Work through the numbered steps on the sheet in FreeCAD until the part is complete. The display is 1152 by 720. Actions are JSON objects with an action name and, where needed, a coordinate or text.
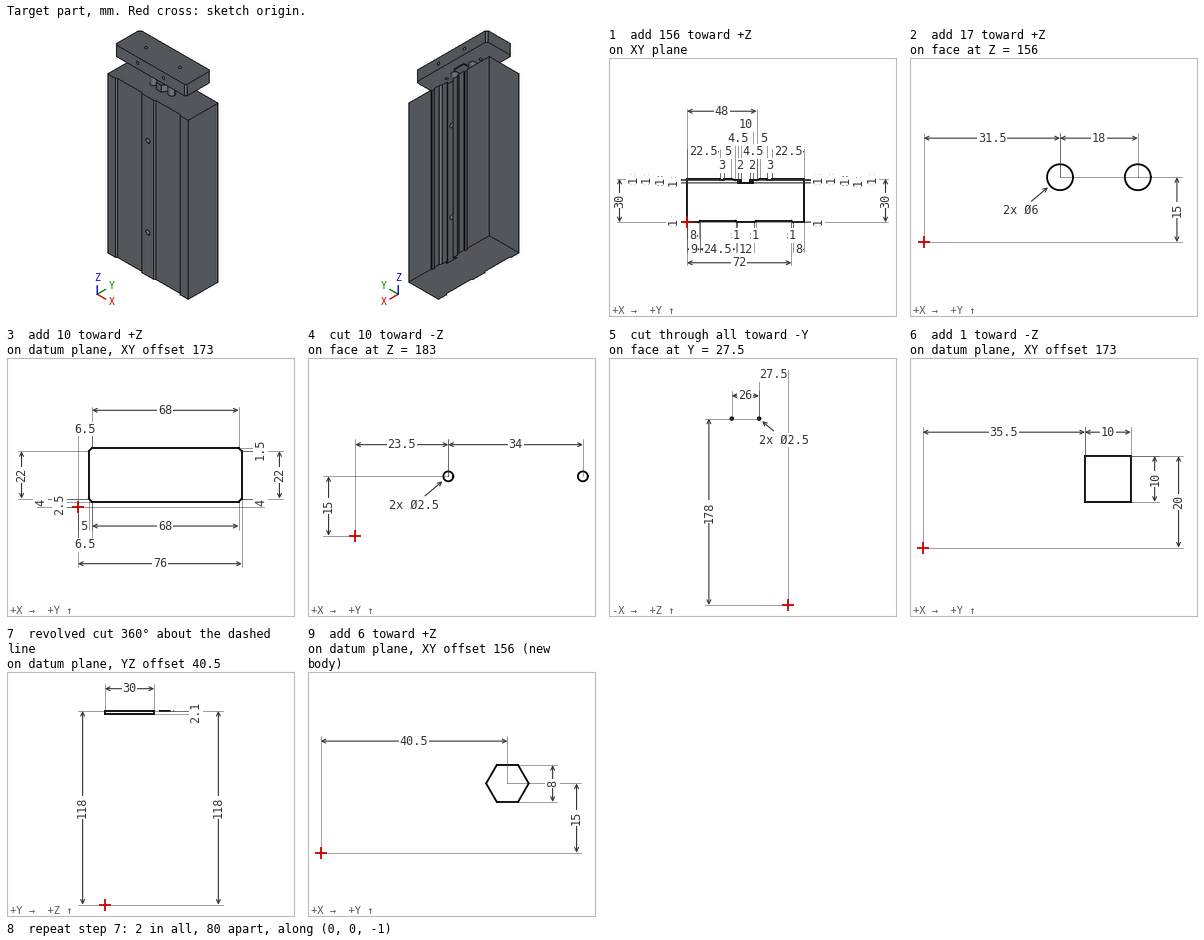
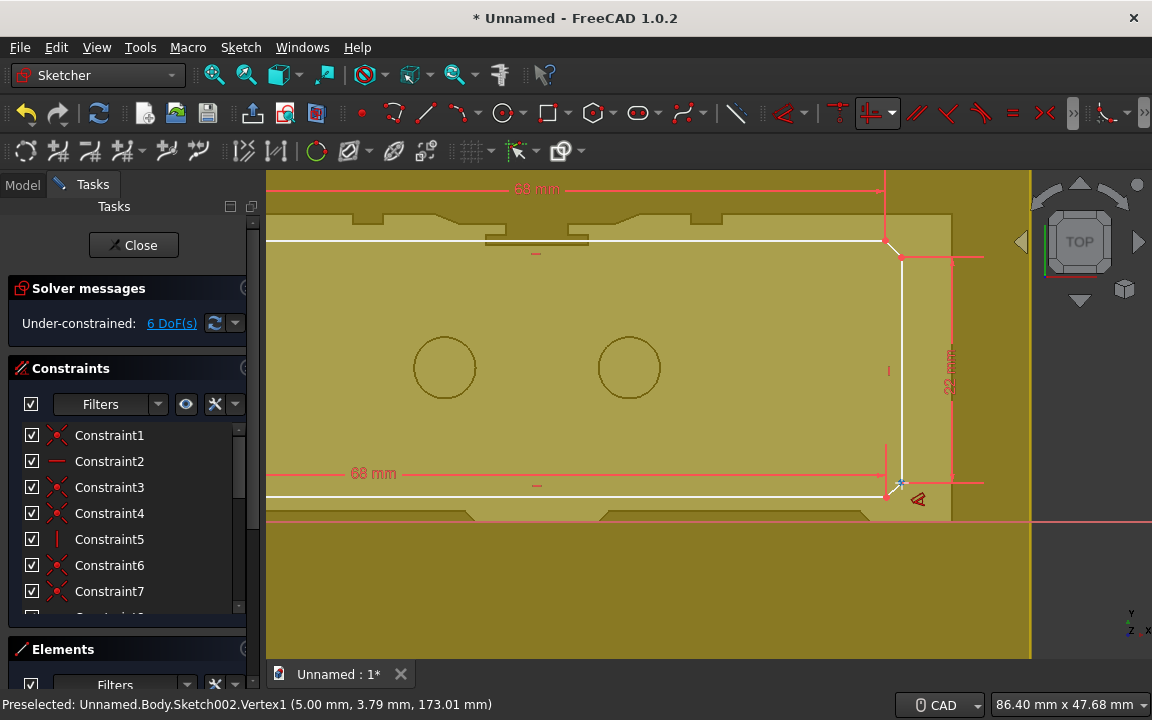
{"action": "left_click", "coordinate": [902, 483]}
{"action": "left_click", "coordinate": [936, 502]}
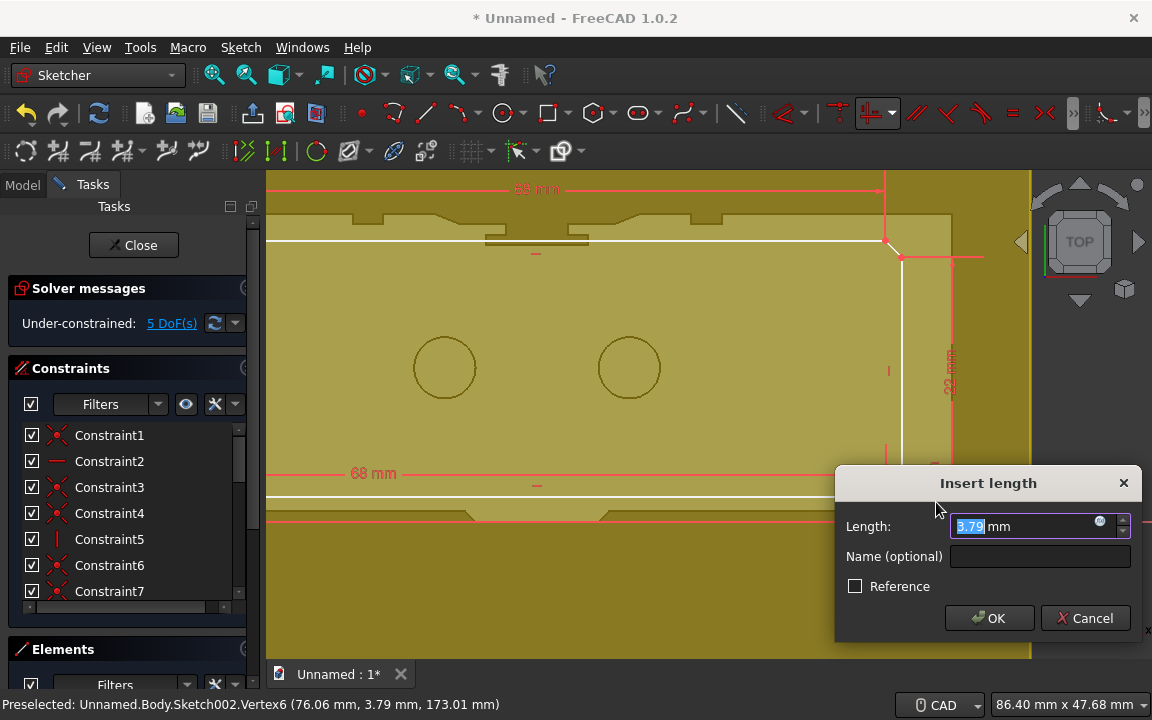
{"action": "type", "text": "4"}
{"action": "key", "text": "Return"}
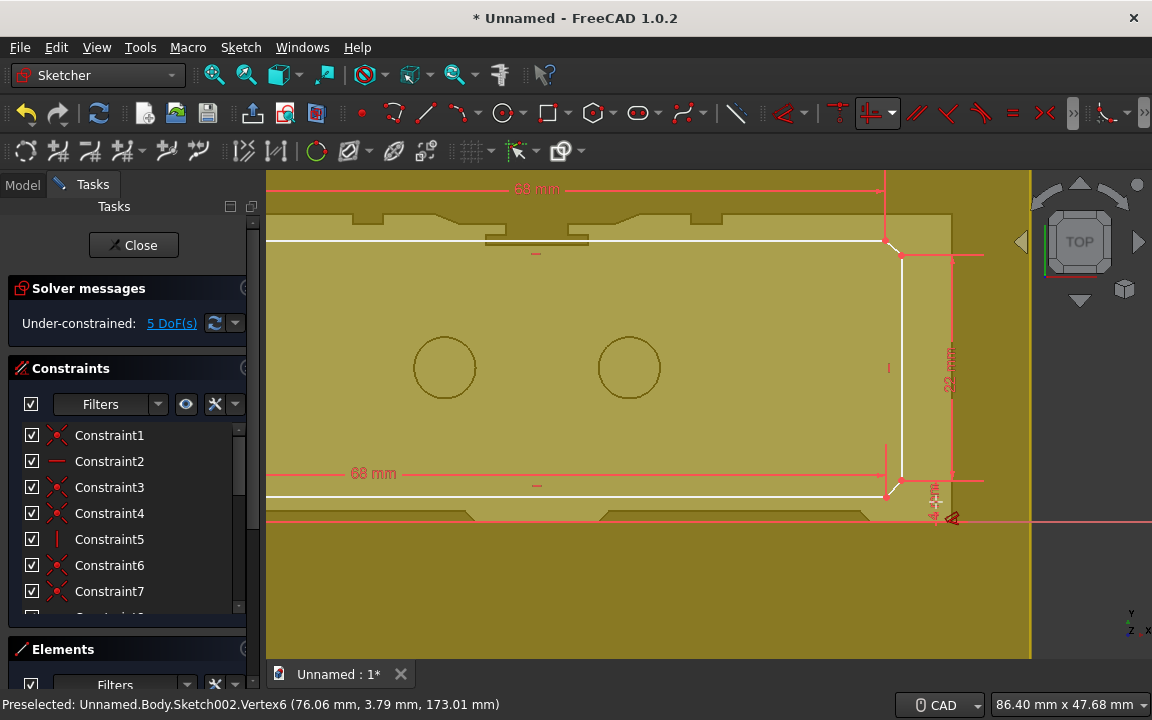
{"action": "left_click", "coordinate": [902, 481]}
{"action": "left_click", "coordinate": [598, 556]}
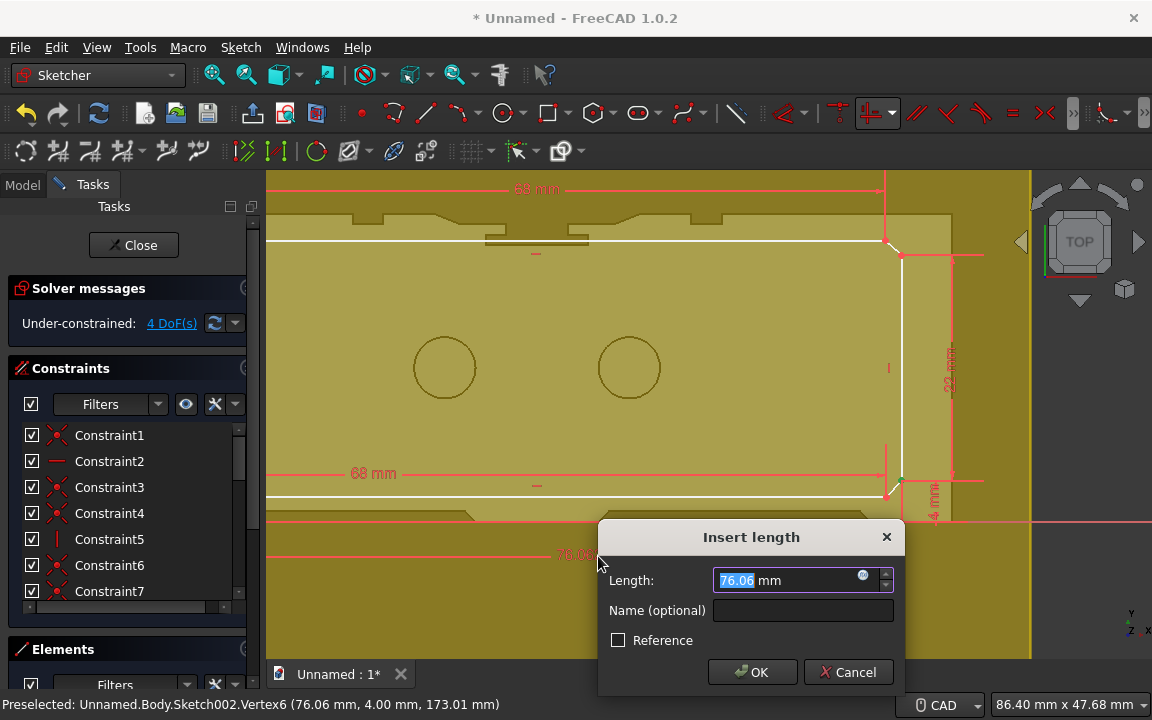
{"action": "type", "text": "76"}
{"action": "key", "text": "Return"}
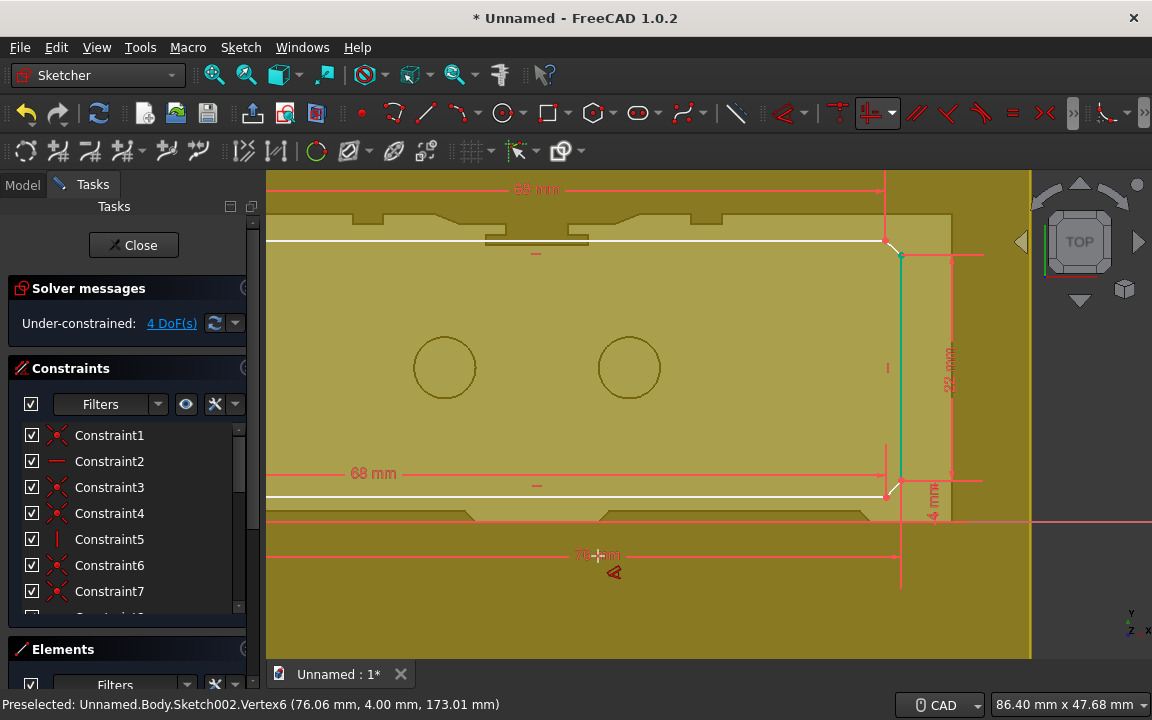
{"action": "scroll", "coordinate": [903, 483], "scroll_direction": "down", "scroll_amount": 2}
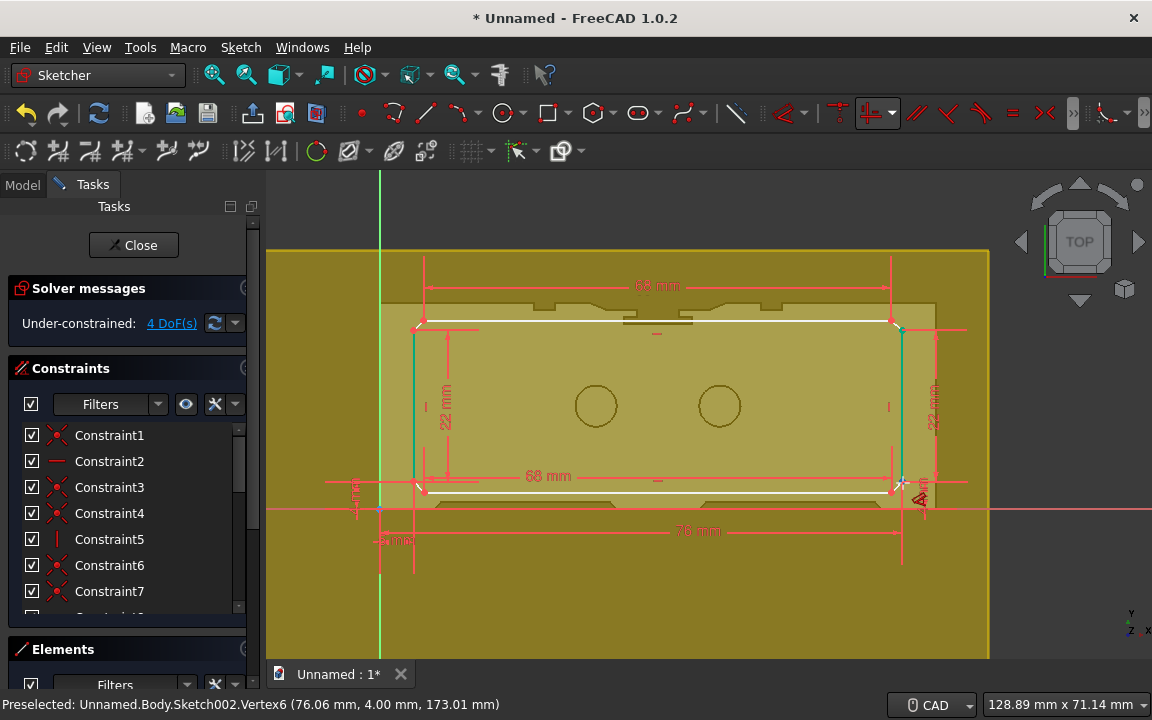
{"action": "left_click", "coordinate": [424, 493]}
{"action": "left_click", "coordinate": [402, 567]}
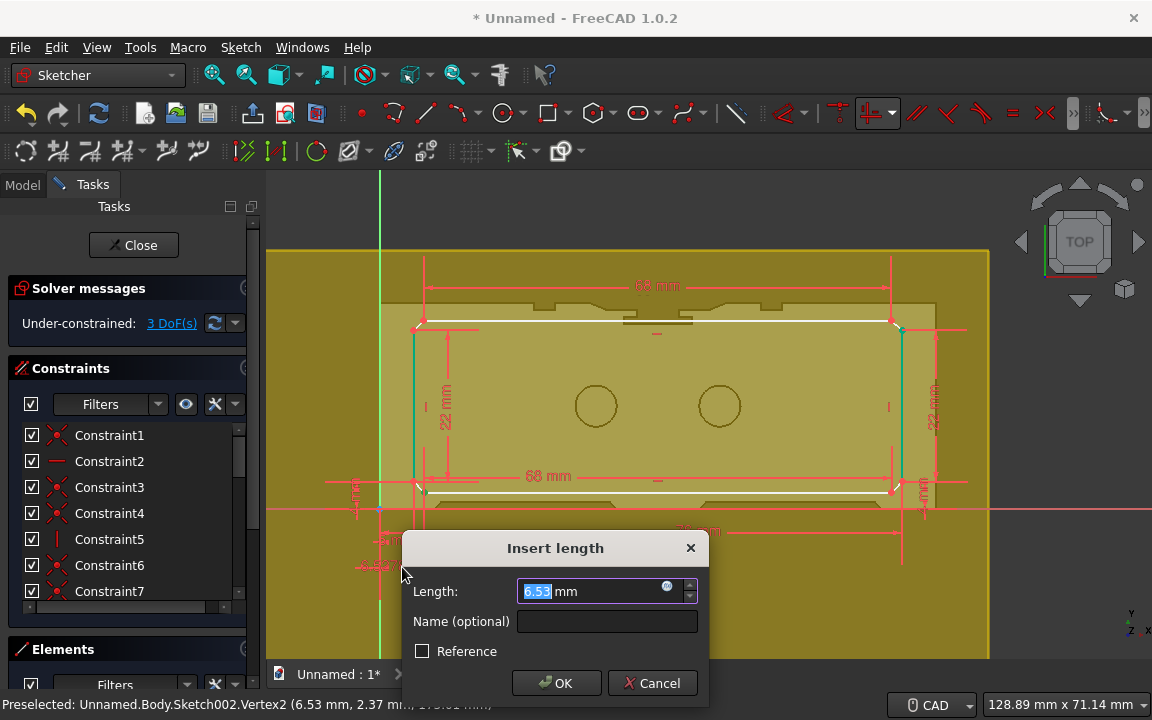
{"action": "type", "text": "6.5"}
{"action": "key", "text": "Return"}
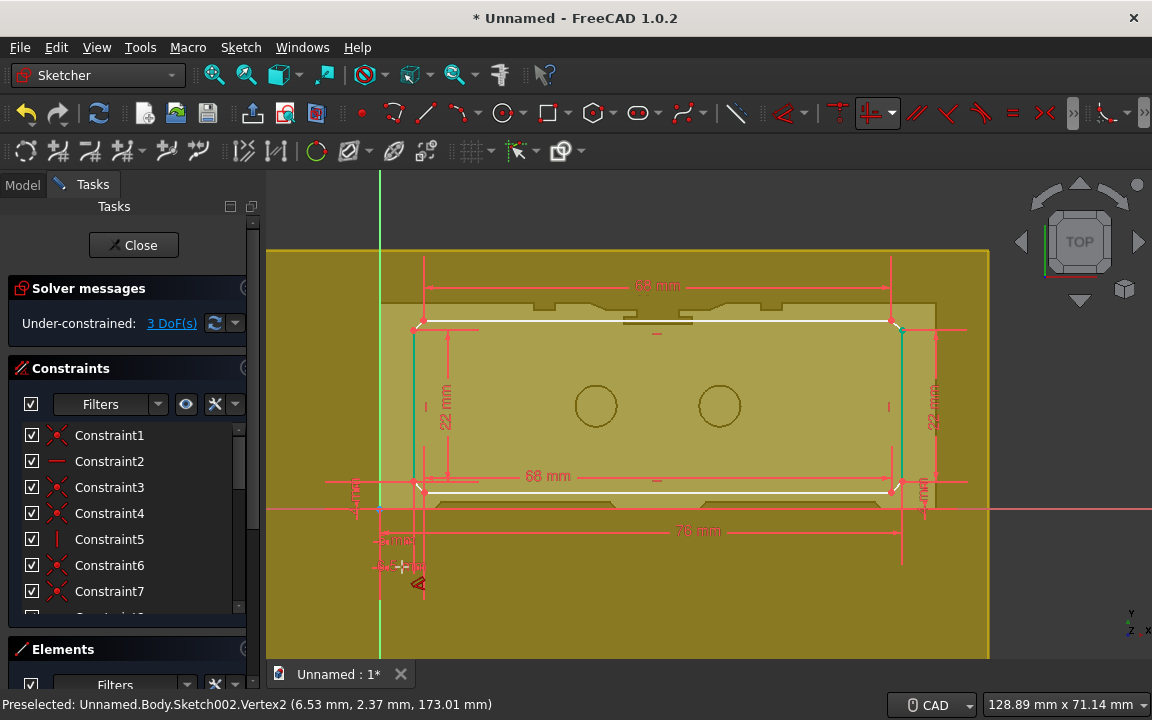
{"action": "scroll", "coordinate": [424, 493], "scroll_direction": "up", "scroll_amount": 5}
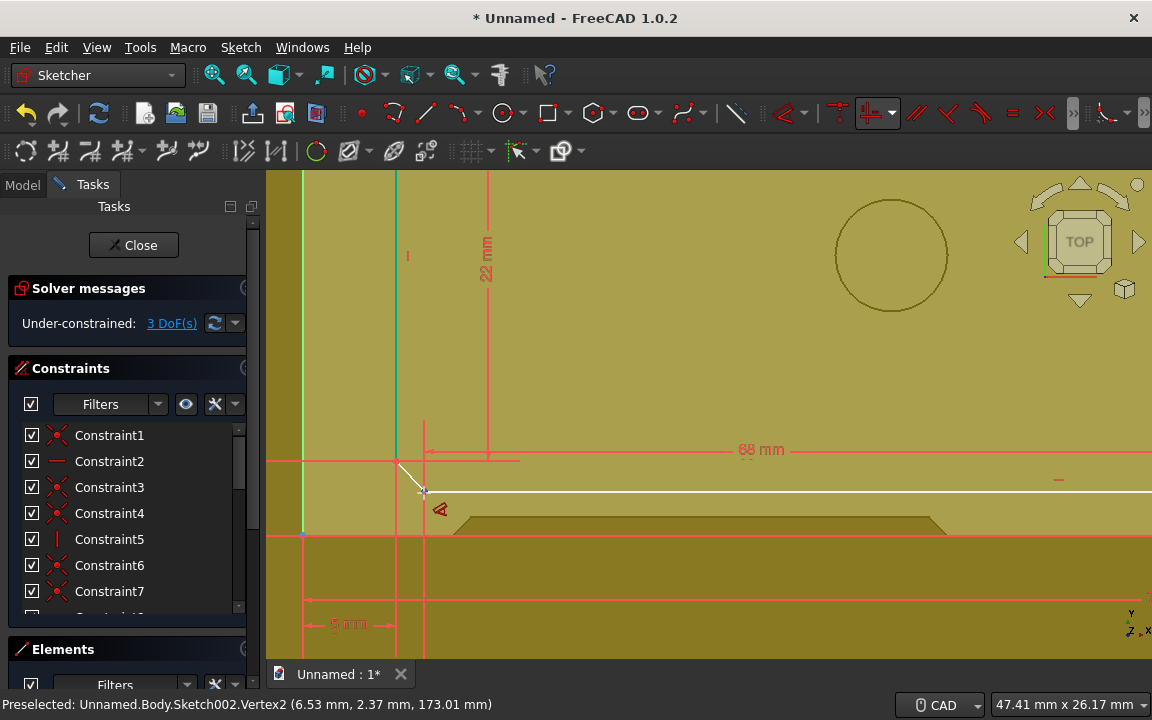
{"action": "left_click", "coordinate": [424, 492]}
{"action": "left_click", "coordinate": [458, 514]}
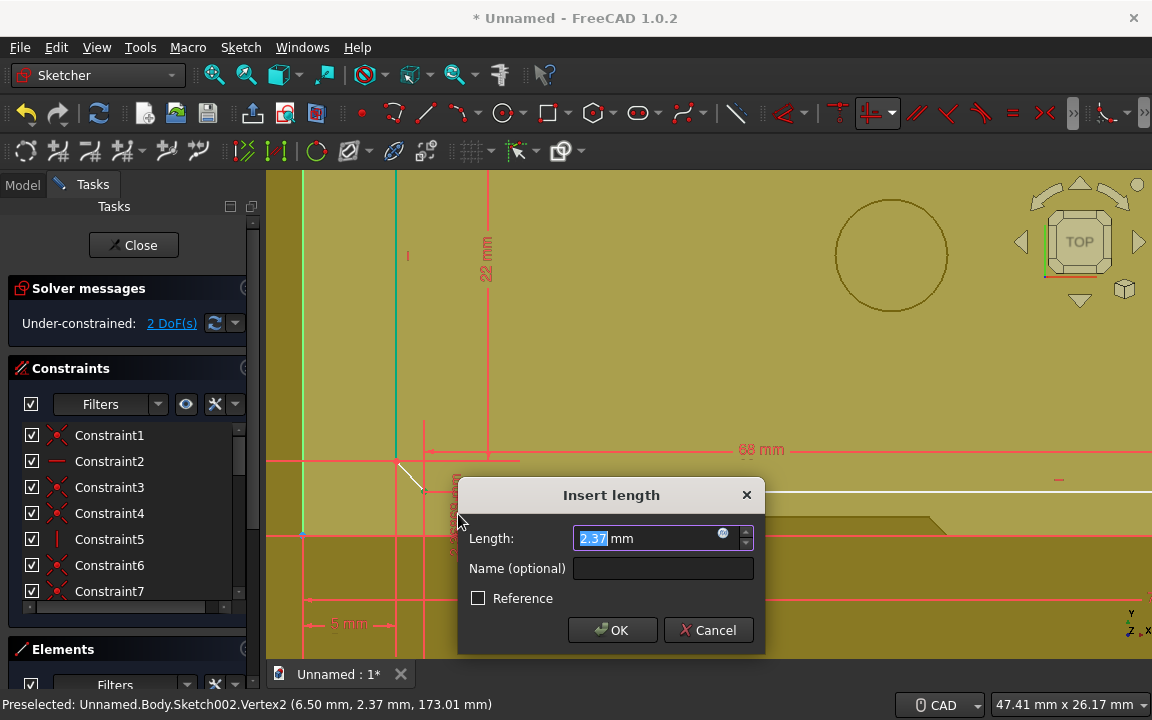
{"action": "type", "text": "2.5"}
{"action": "key", "text": "Return"}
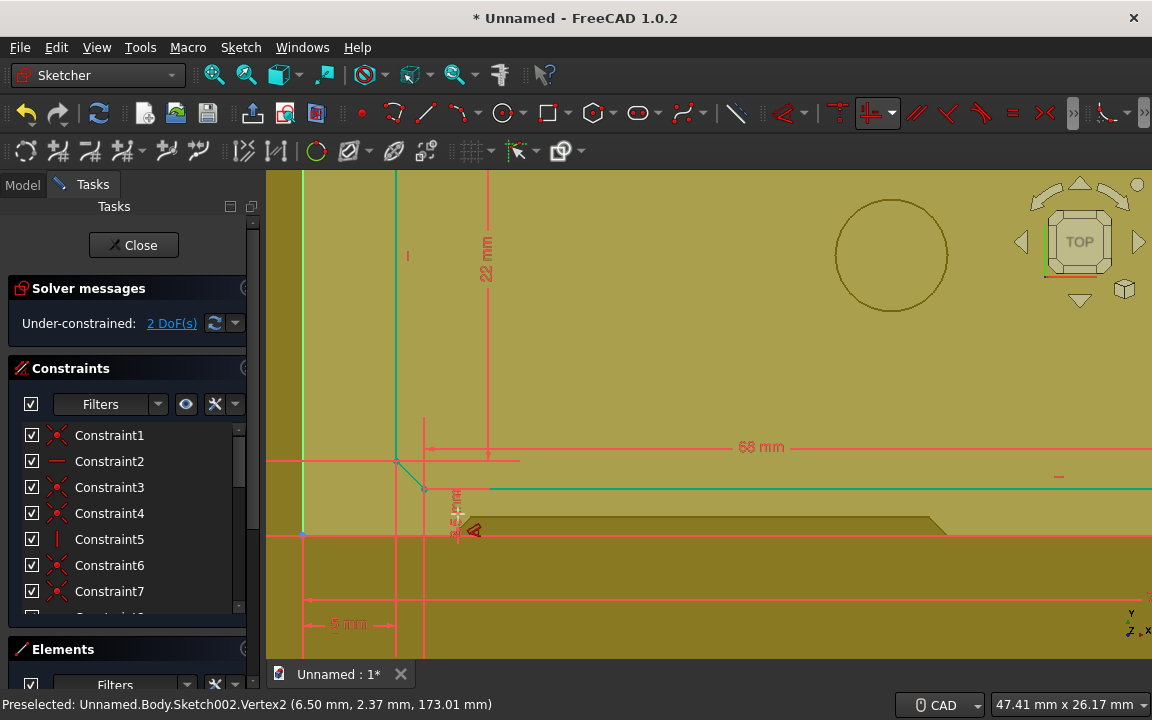
{"action": "scroll", "coordinate": [424, 493], "scroll_direction": "down", "scroll_amount": 5}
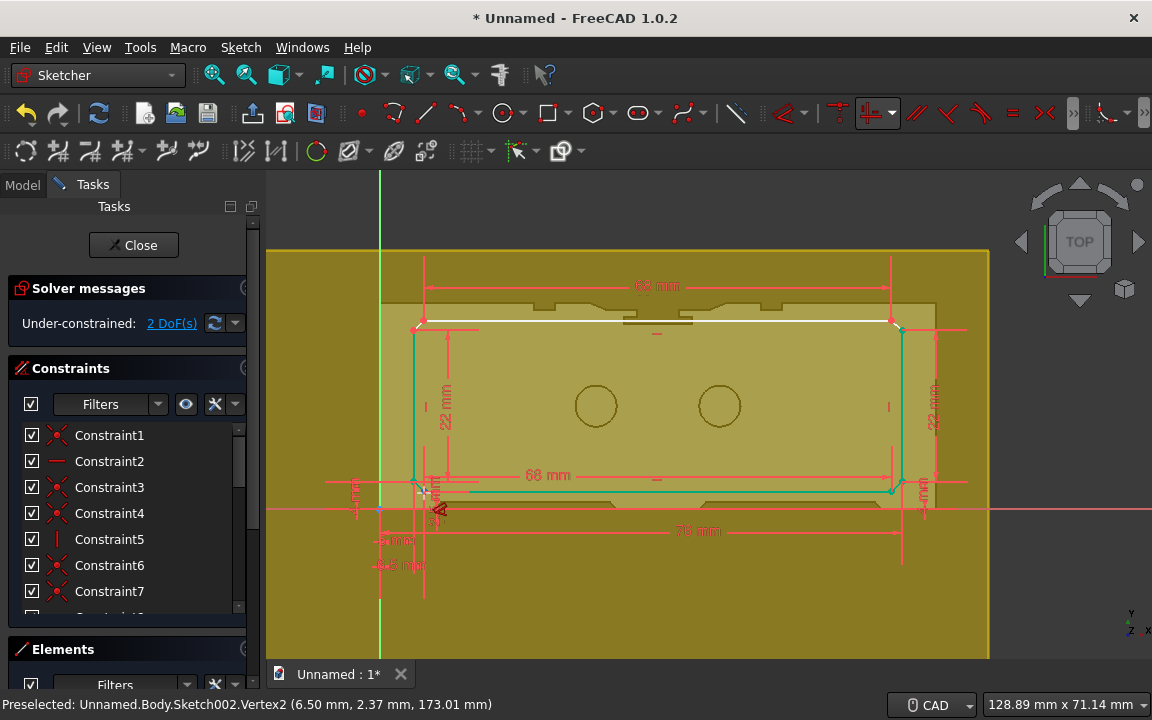
{"action": "left_click", "coordinate": [424, 321]}
{"action": "left_click", "coordinate": [402, 287]}